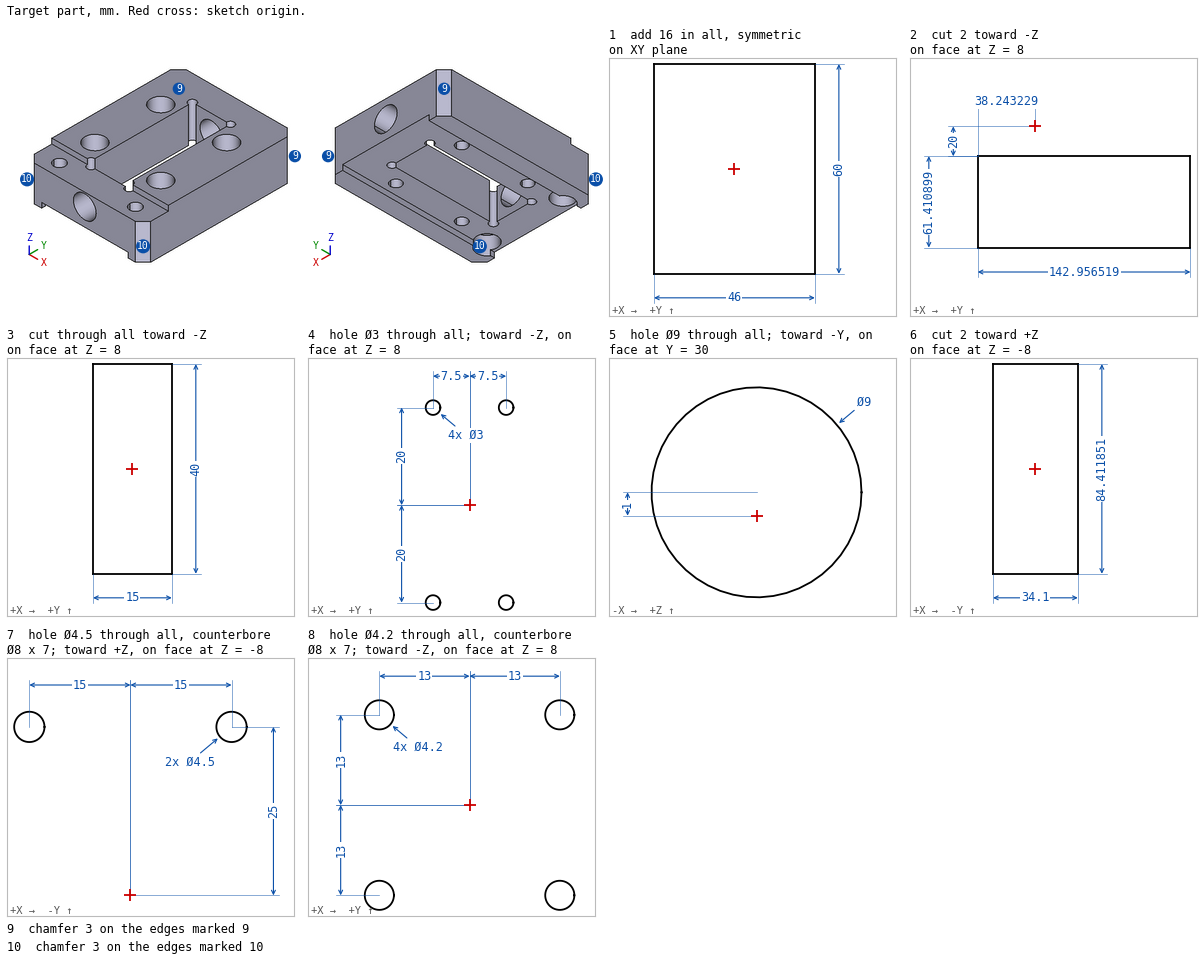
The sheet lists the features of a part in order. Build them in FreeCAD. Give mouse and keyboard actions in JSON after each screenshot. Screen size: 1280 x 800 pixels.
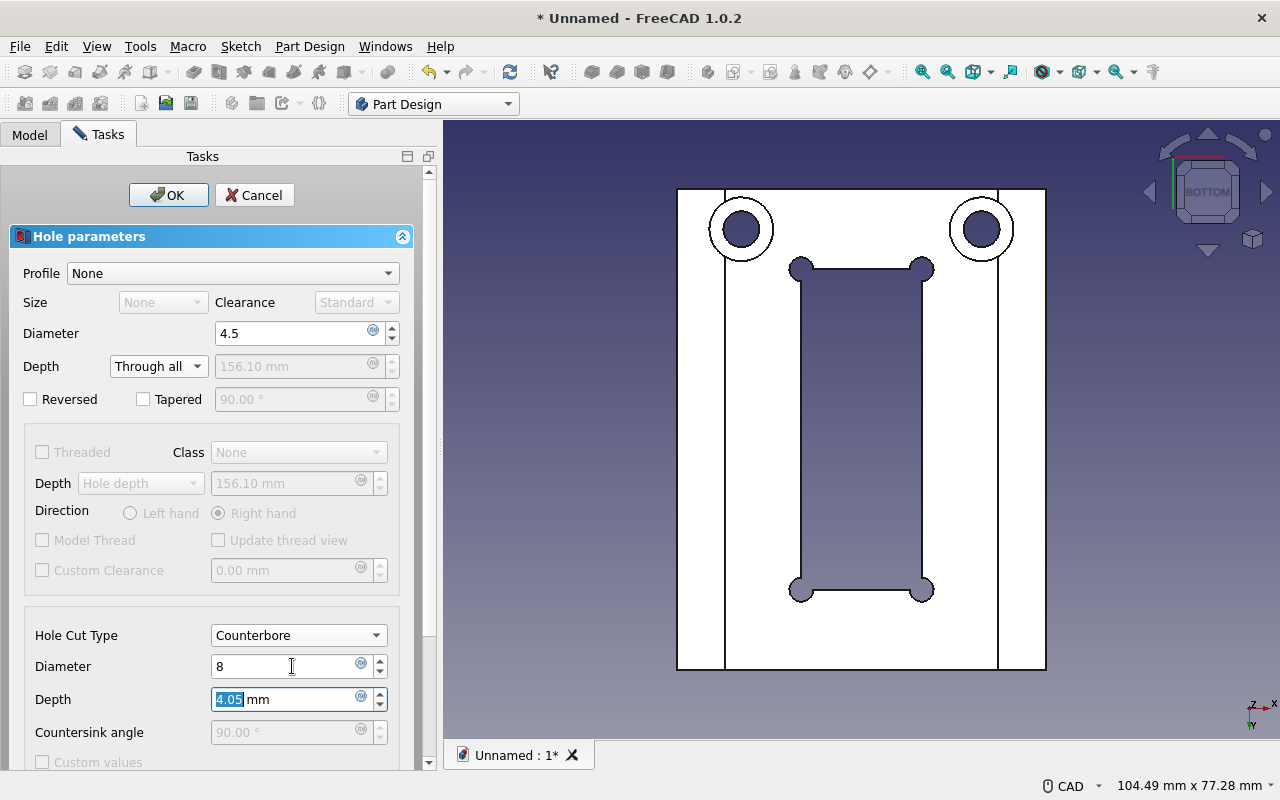
{"action": "type", "text": "7"}
{"action": "key", "text": "Tab"}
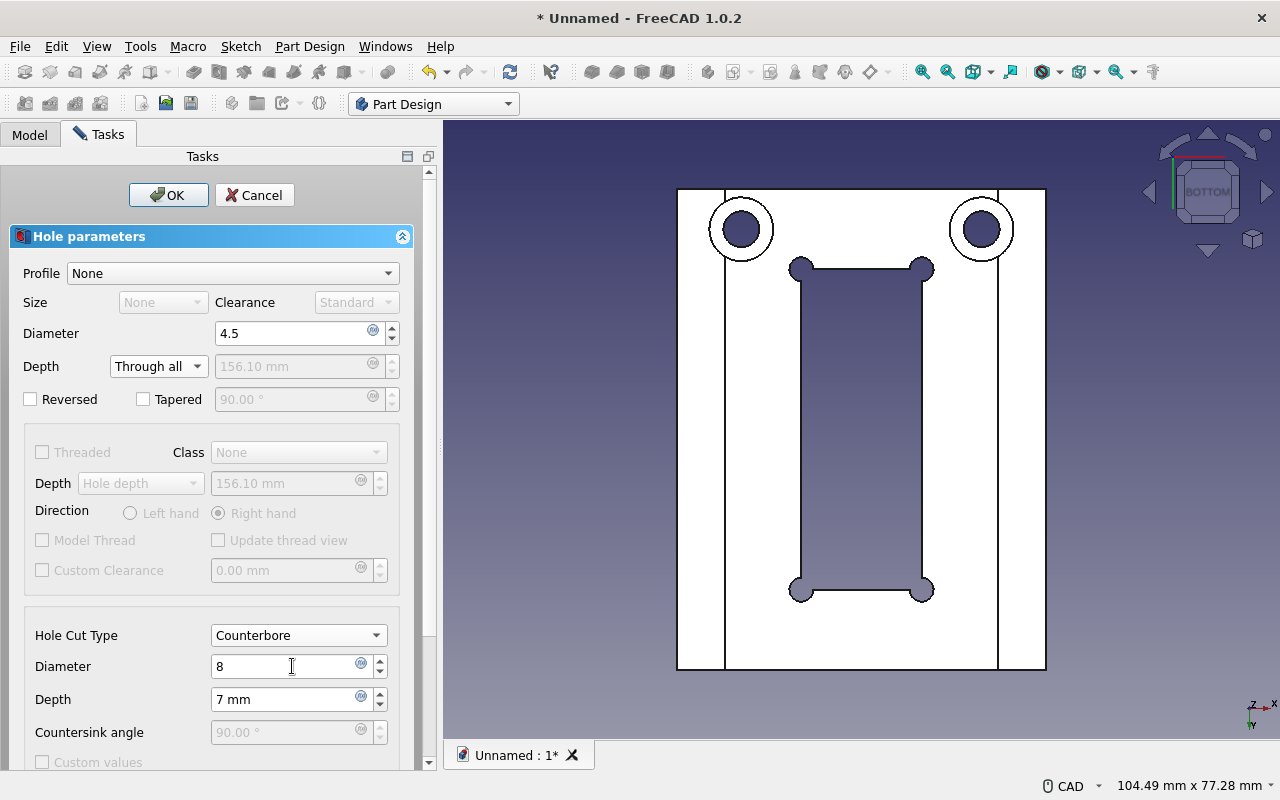
{"action": "left_click", "coordinate": [169, 195]}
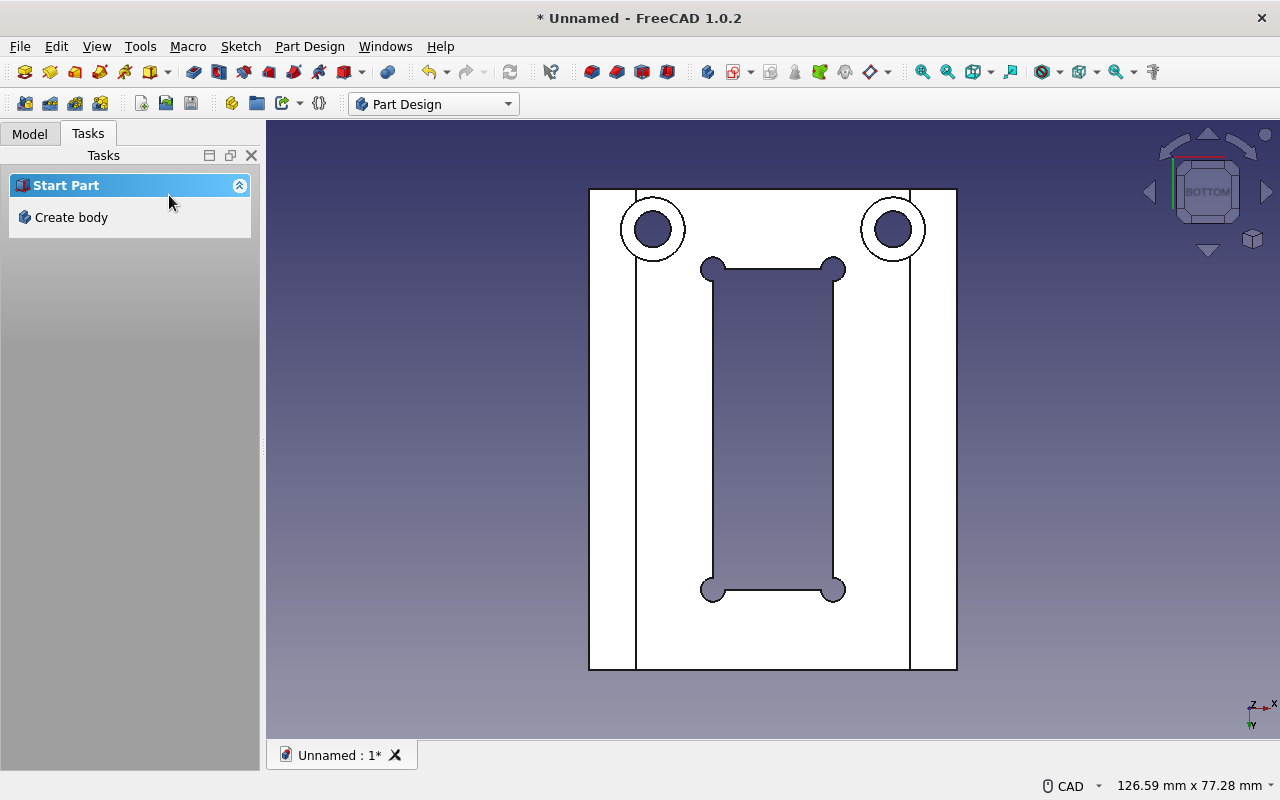
{"action": "key", "text": "0"}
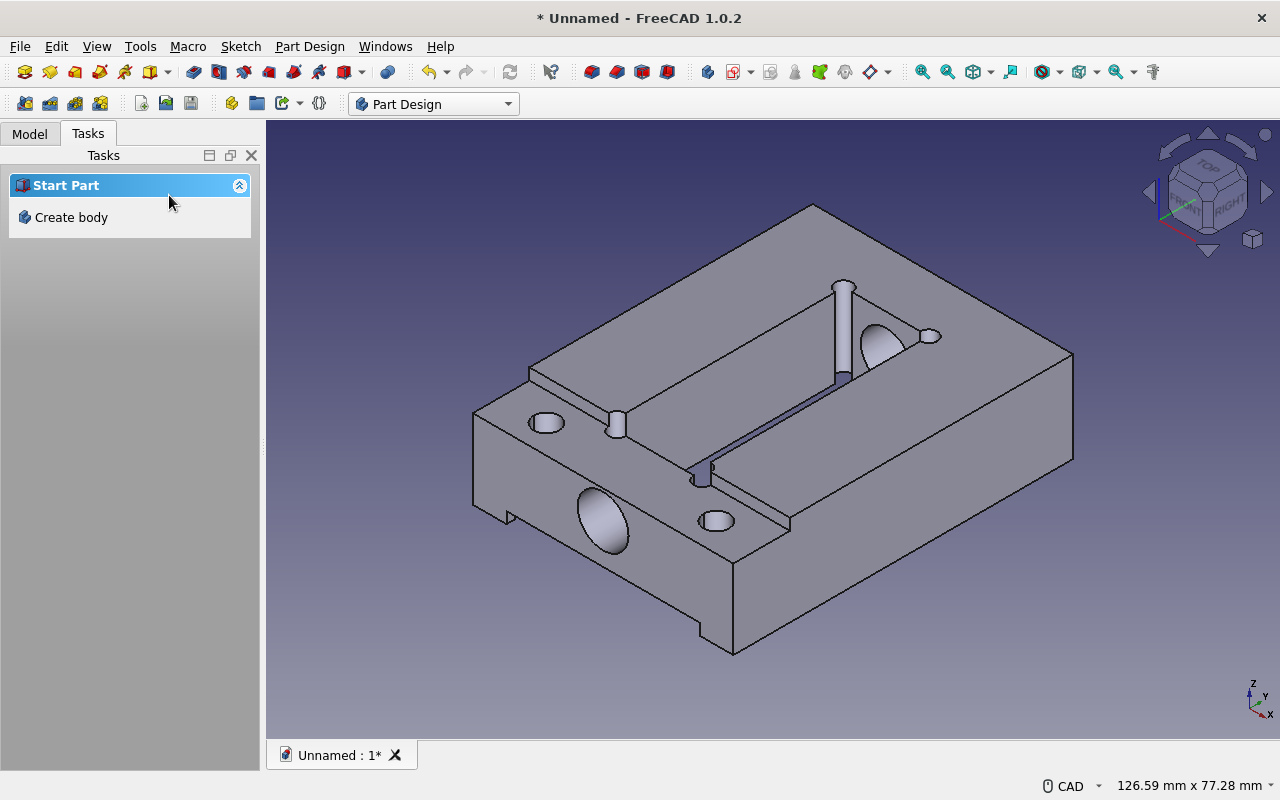
{"action": "left_click", "coordinate": [916, 379]}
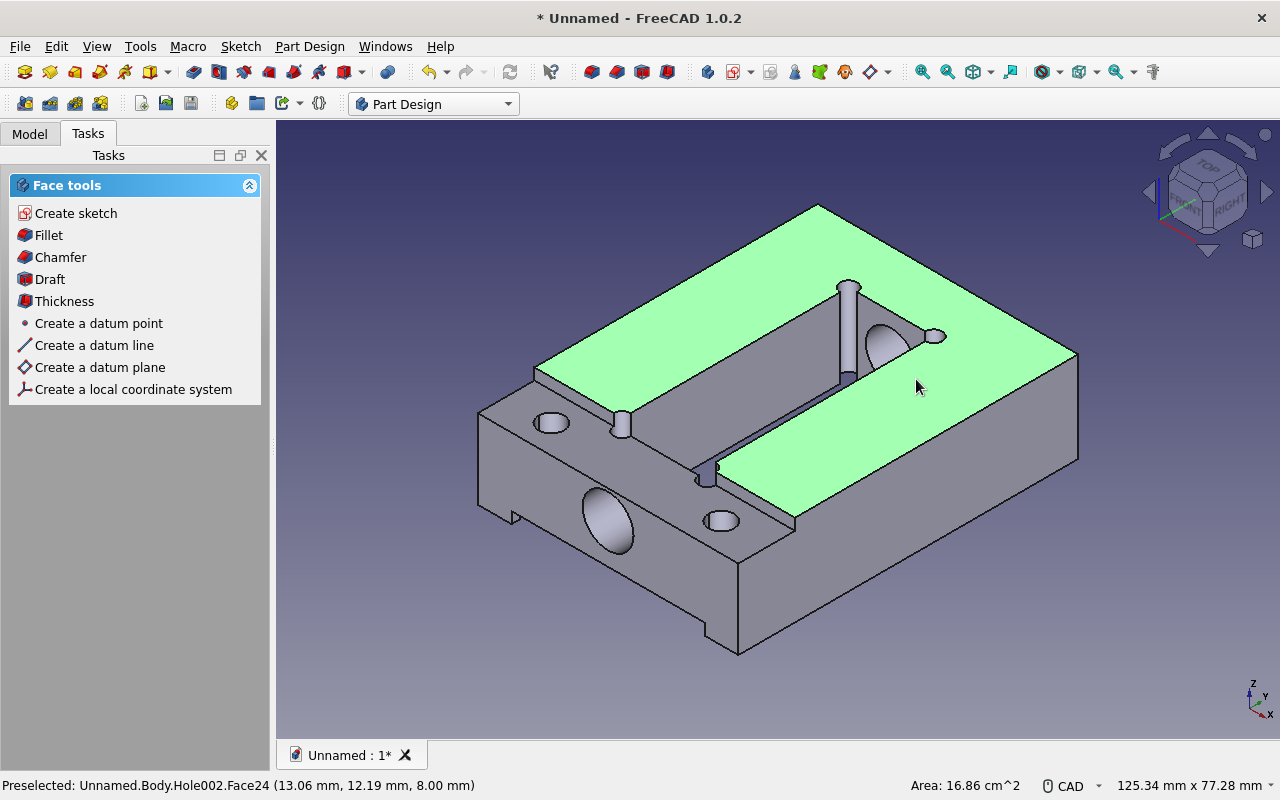
{"action": "left_click", "coordinate": [732, 72]}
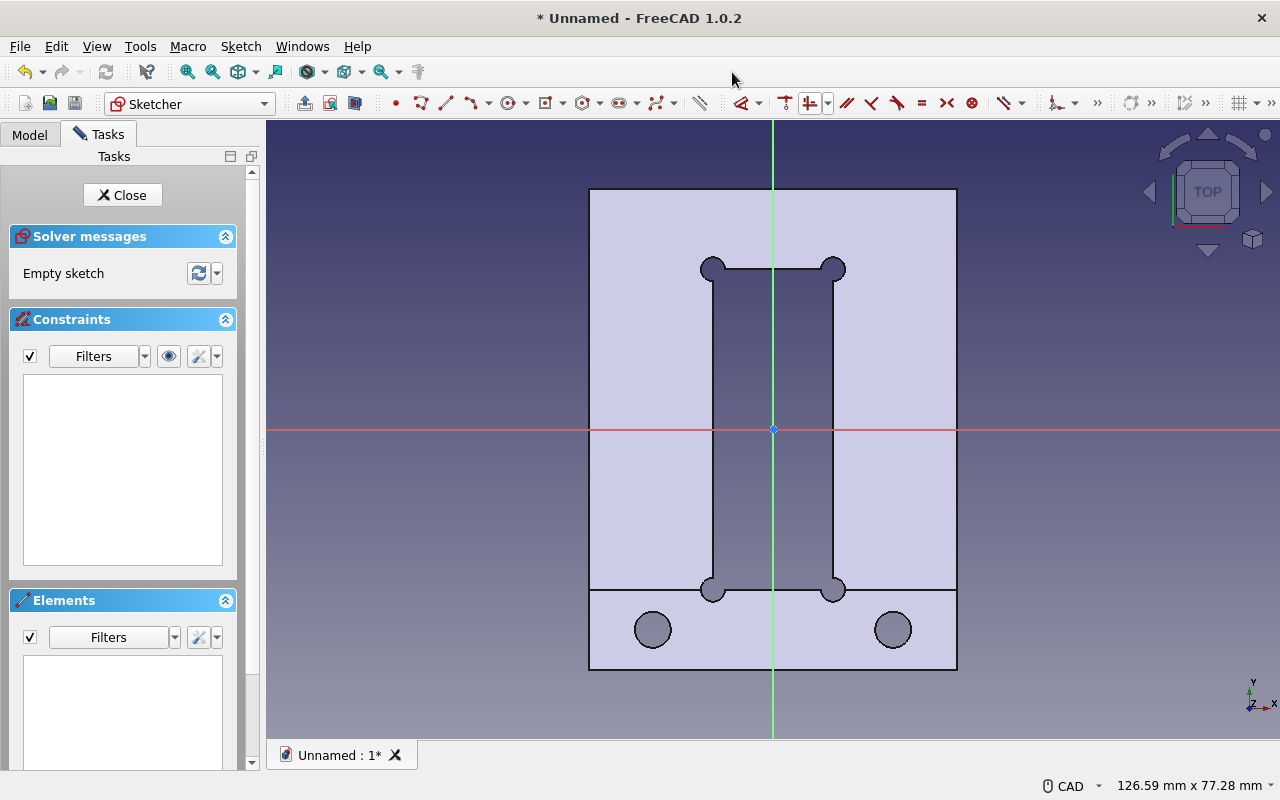
{"action": "scroll", "coordinate": [912, 429], "scroll_direction": "up", "scroll_amount": 2}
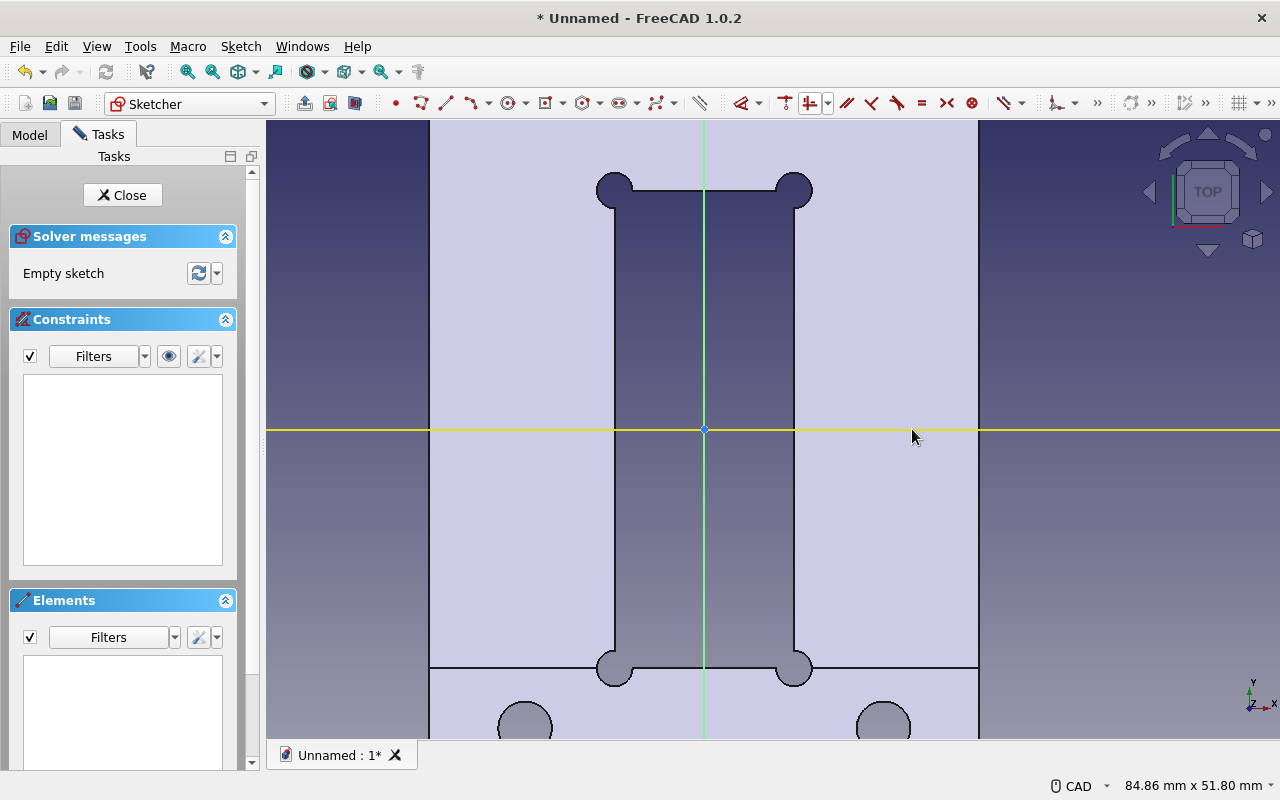
{"action": "left_click", "coordinate": [508, 104]}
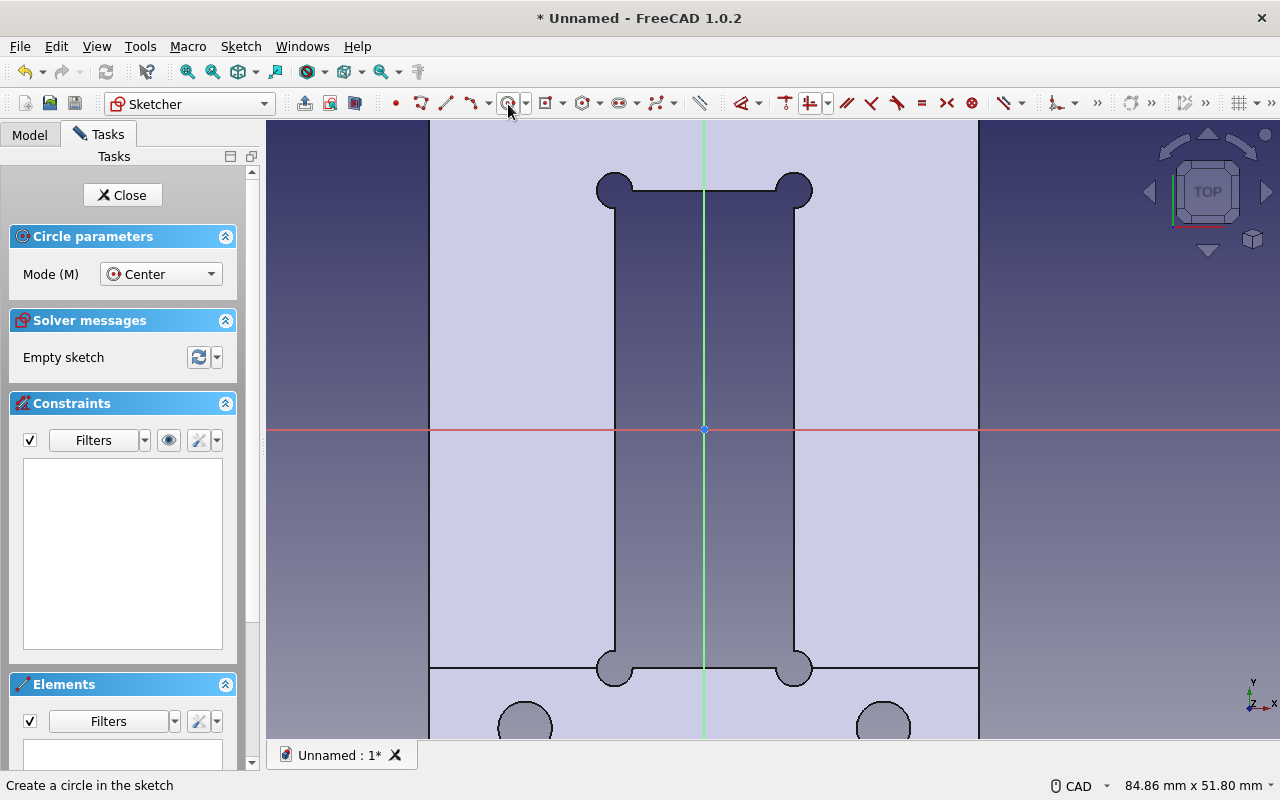
{"action": "left_click", "coordinate": [549, 274]}
{"action": "left_click", "coordinate": [567, 256]}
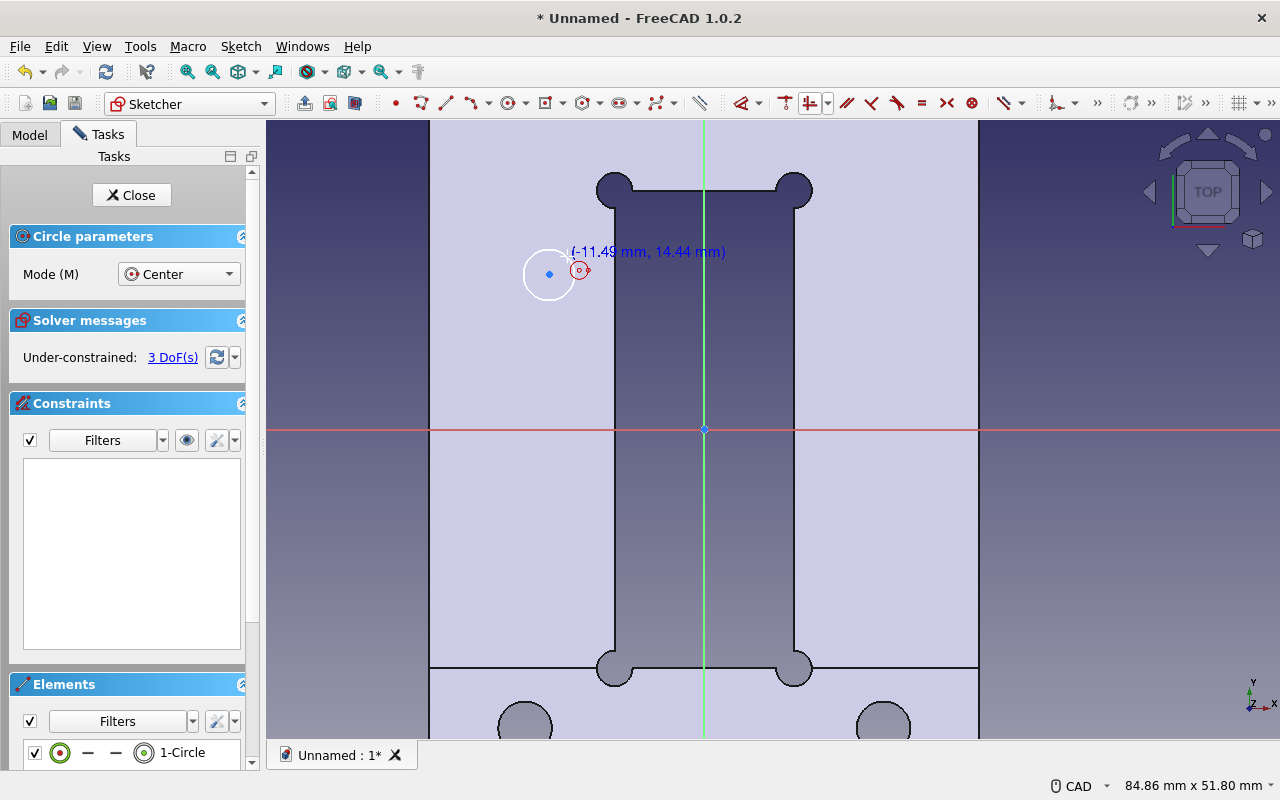
{"action": "left_click", "coordinate": [860, 274]}
{"action": "left_click", "coordinate": [877, 256]}